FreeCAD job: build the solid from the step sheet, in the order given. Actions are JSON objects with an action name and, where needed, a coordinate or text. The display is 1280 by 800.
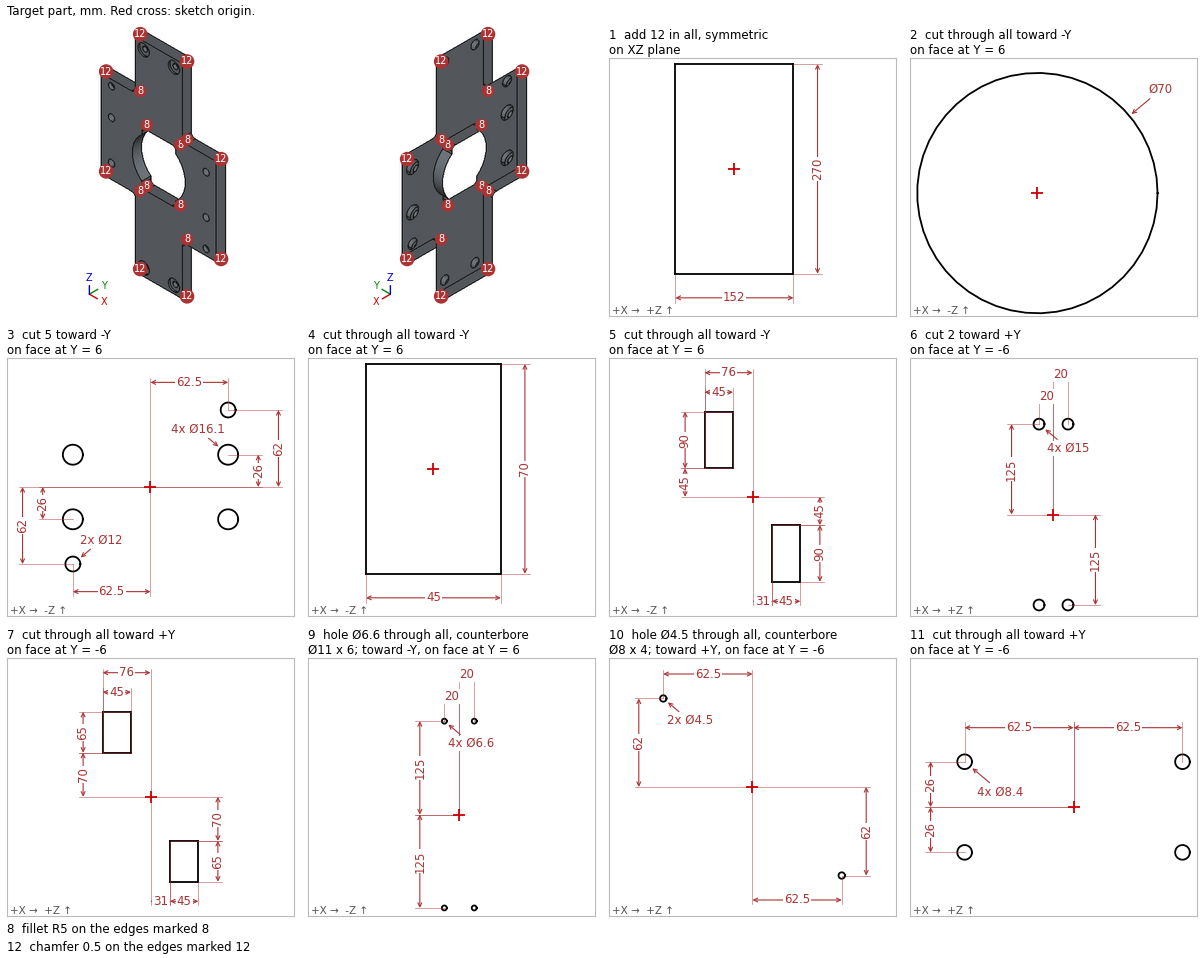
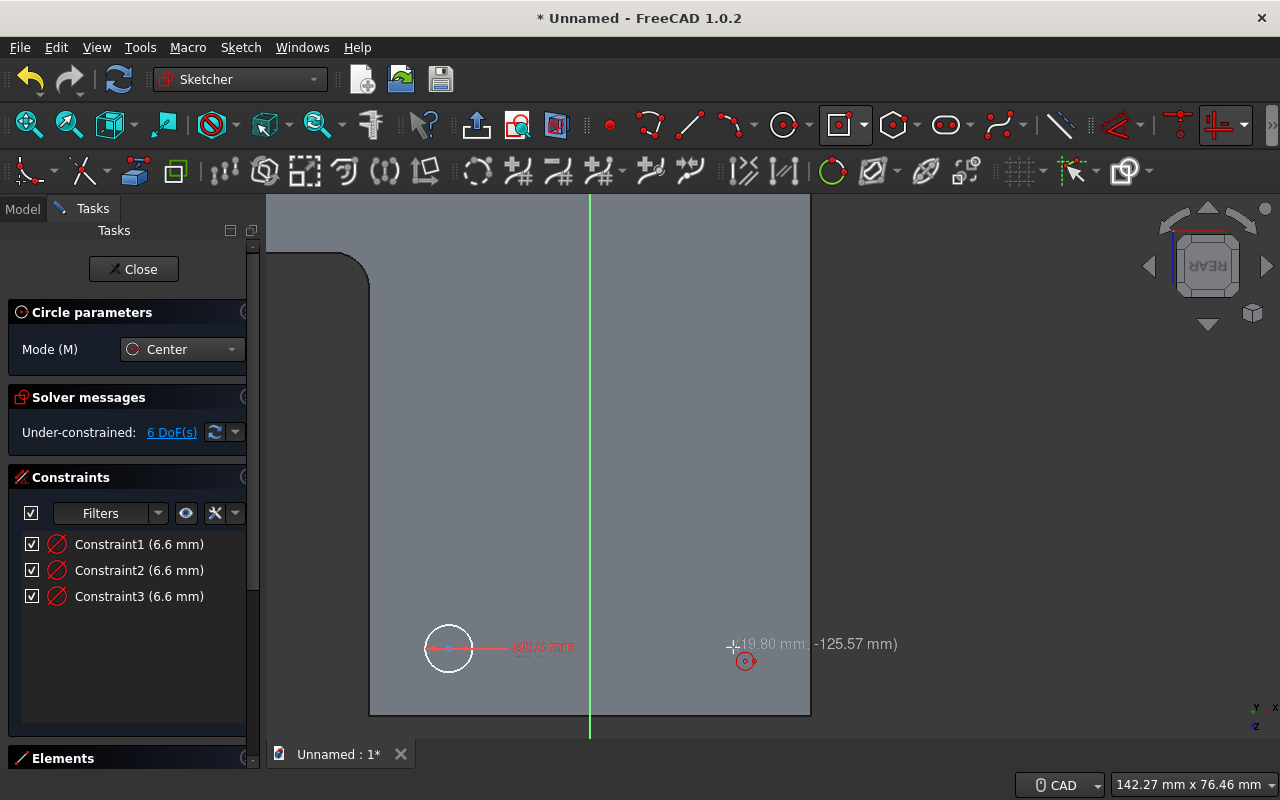
{"action": "scroll", "coordinate": [733, 647], "scroll_direction": "down", "scroll_amount": 8}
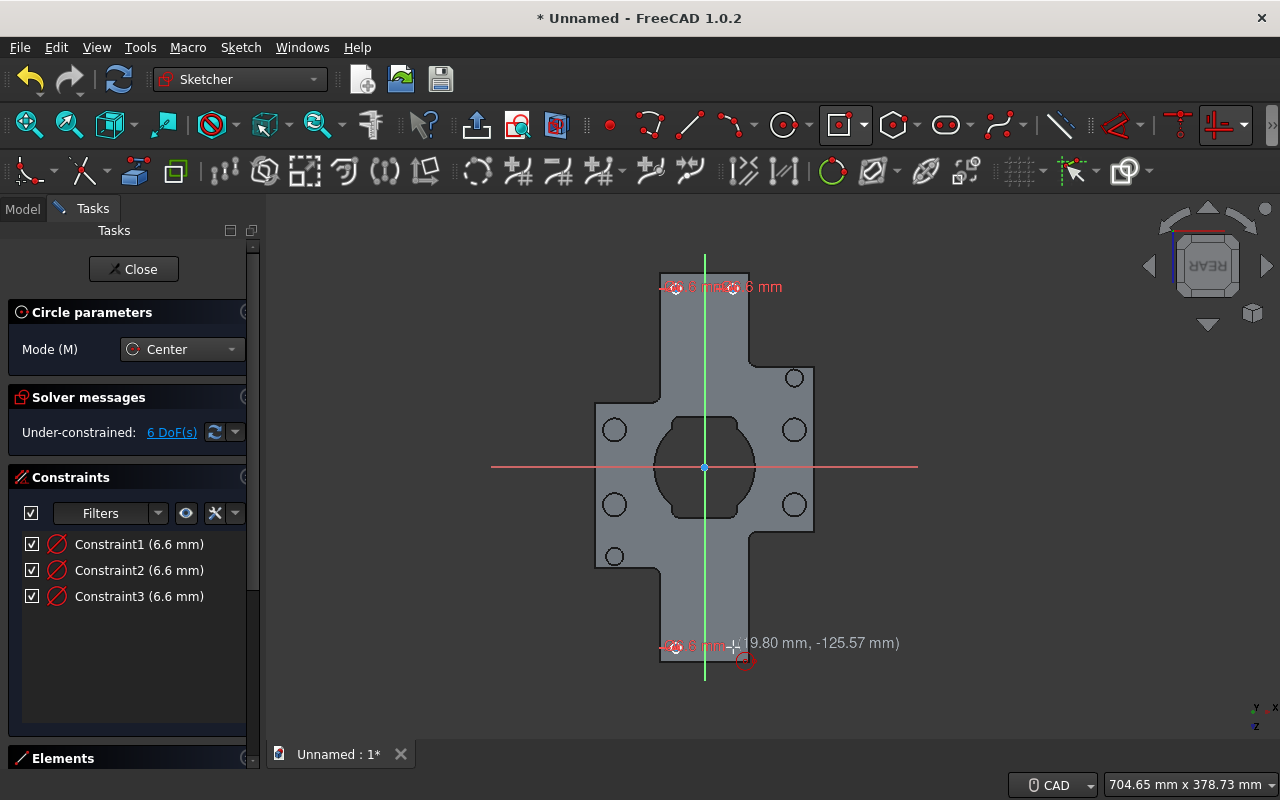
{"action": "left_click", "coordinate": [733, 647]}
{"action": "mouse_move", "coordinate": [737, 644]}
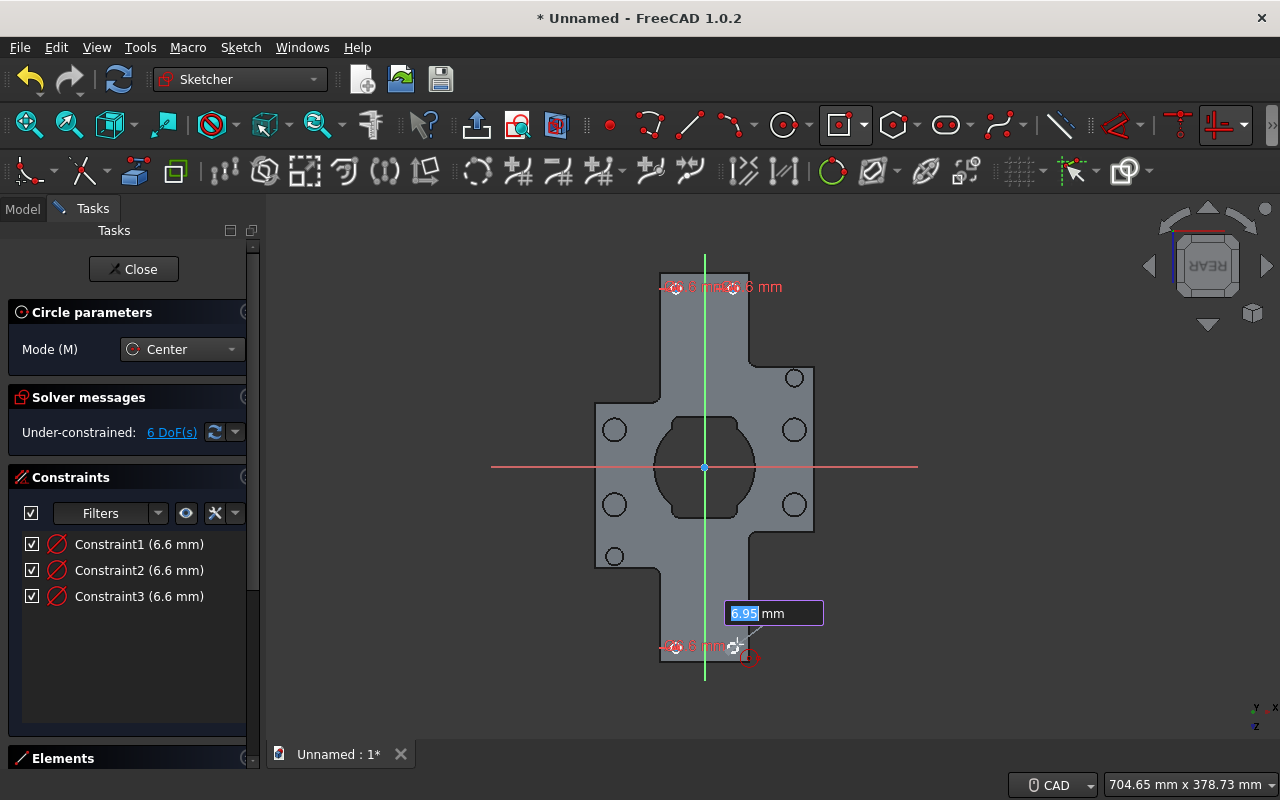
{"action": "type", "text": "6.6"}
{"action": "key", "text": "Return"}
{"action": "key", "text": "Escape"}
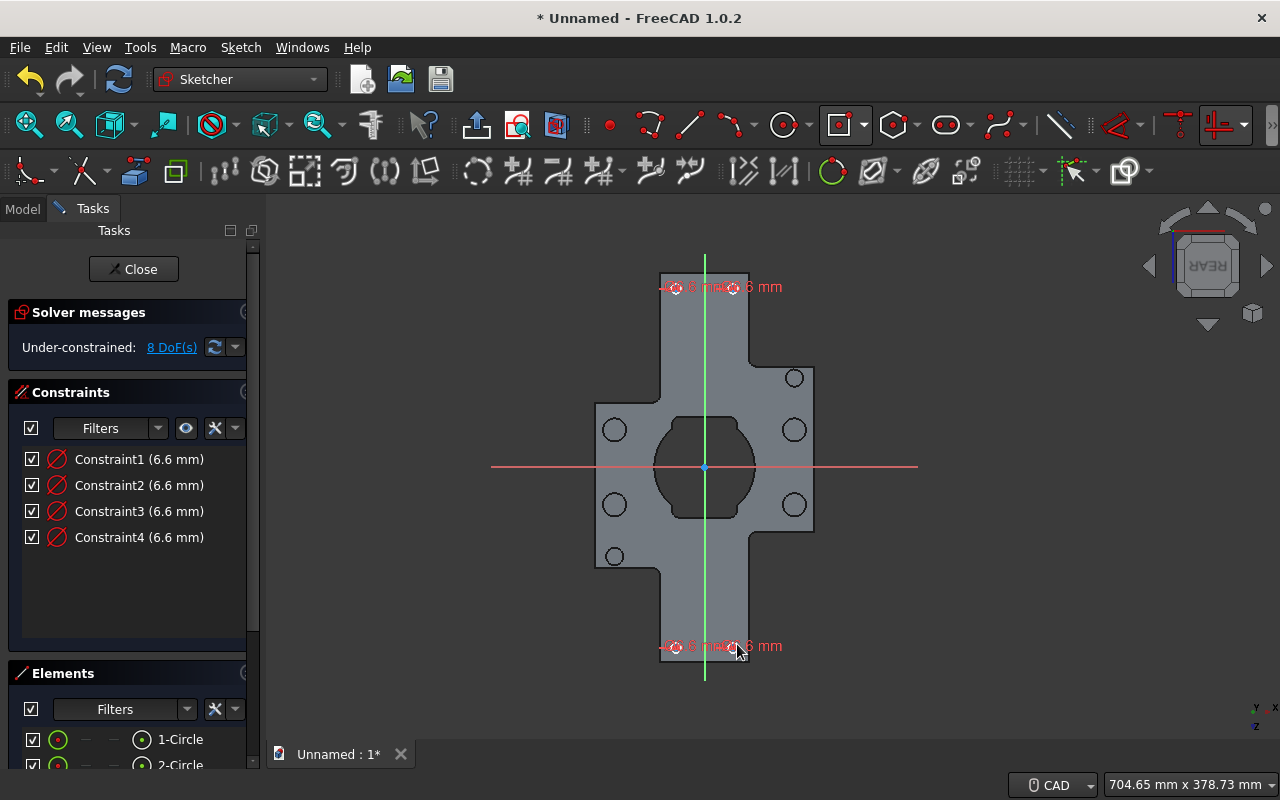
{"action": "left_click", "coordinate": [676, 289]}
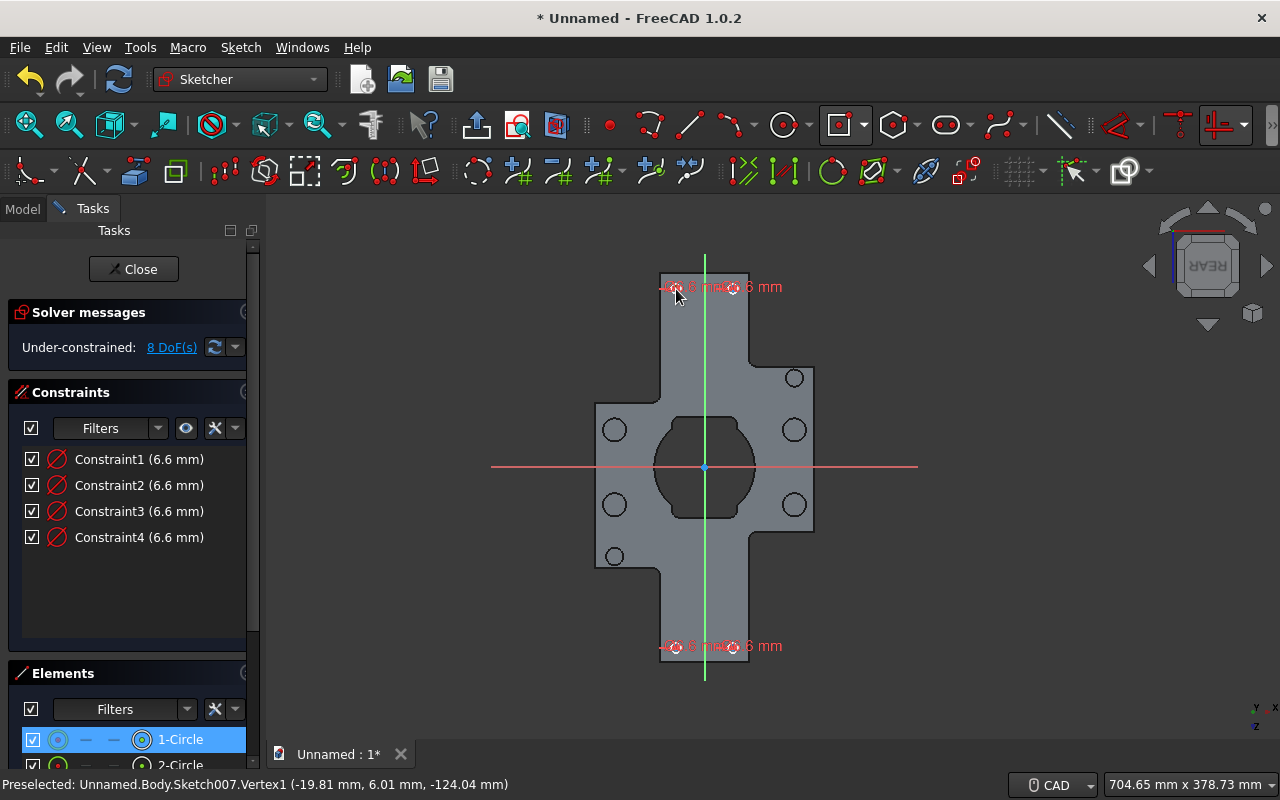
{"action": "left_click", "coordinate": [733, 289]}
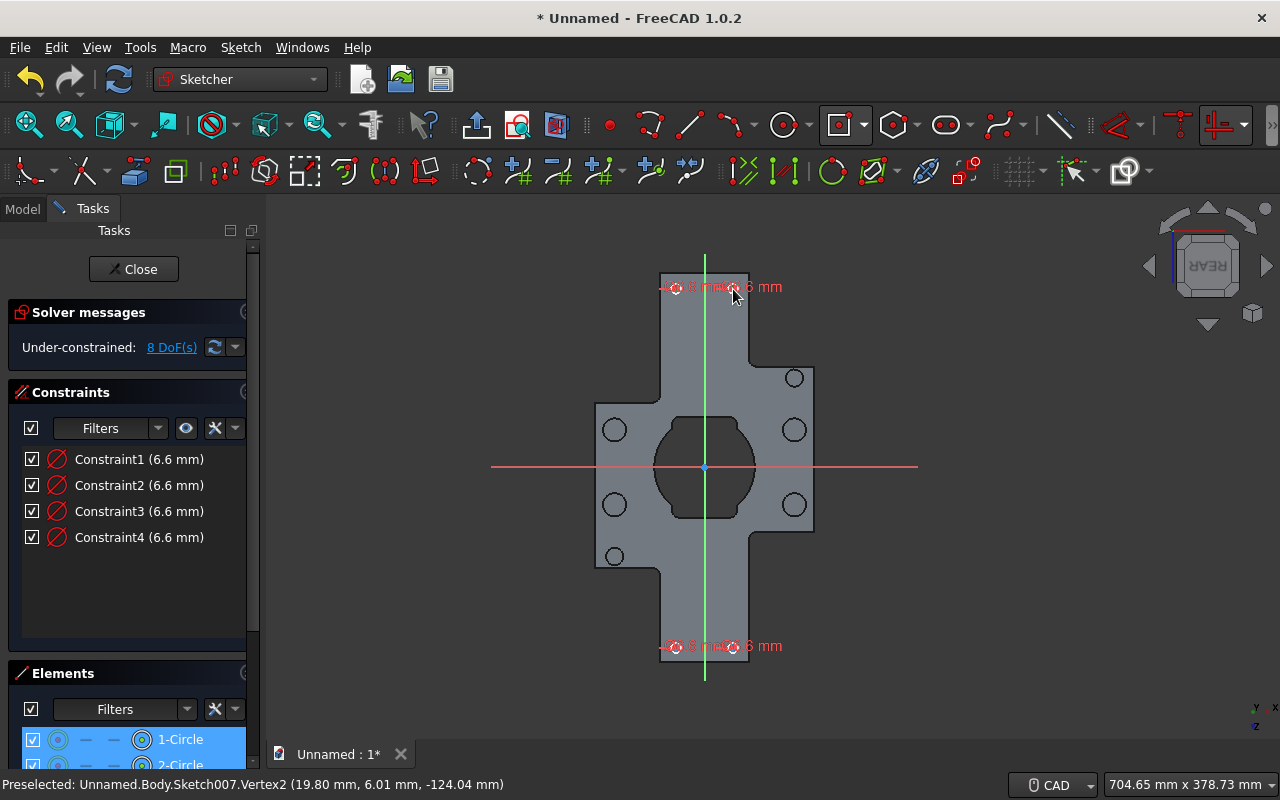
{"action": "key", "text": "h"}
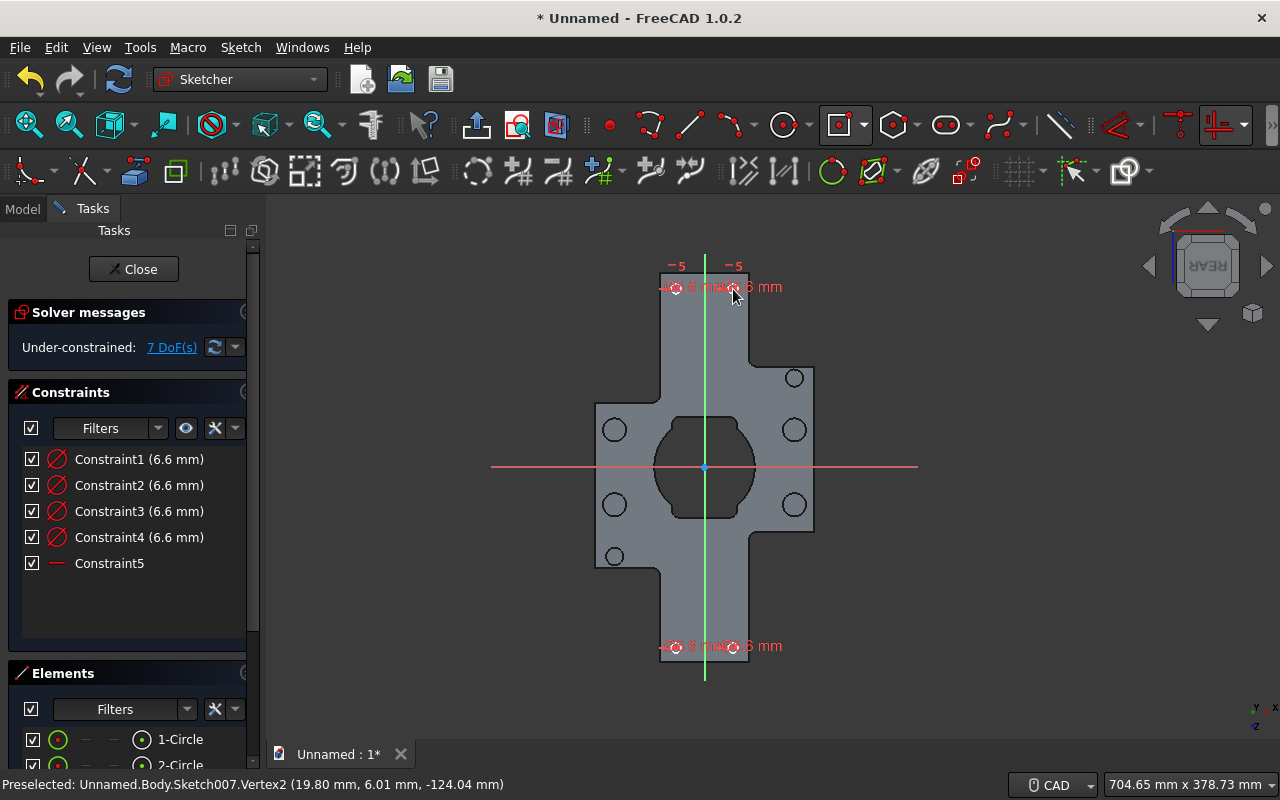
{"action": "left_click", "coordinate": [676, 289]}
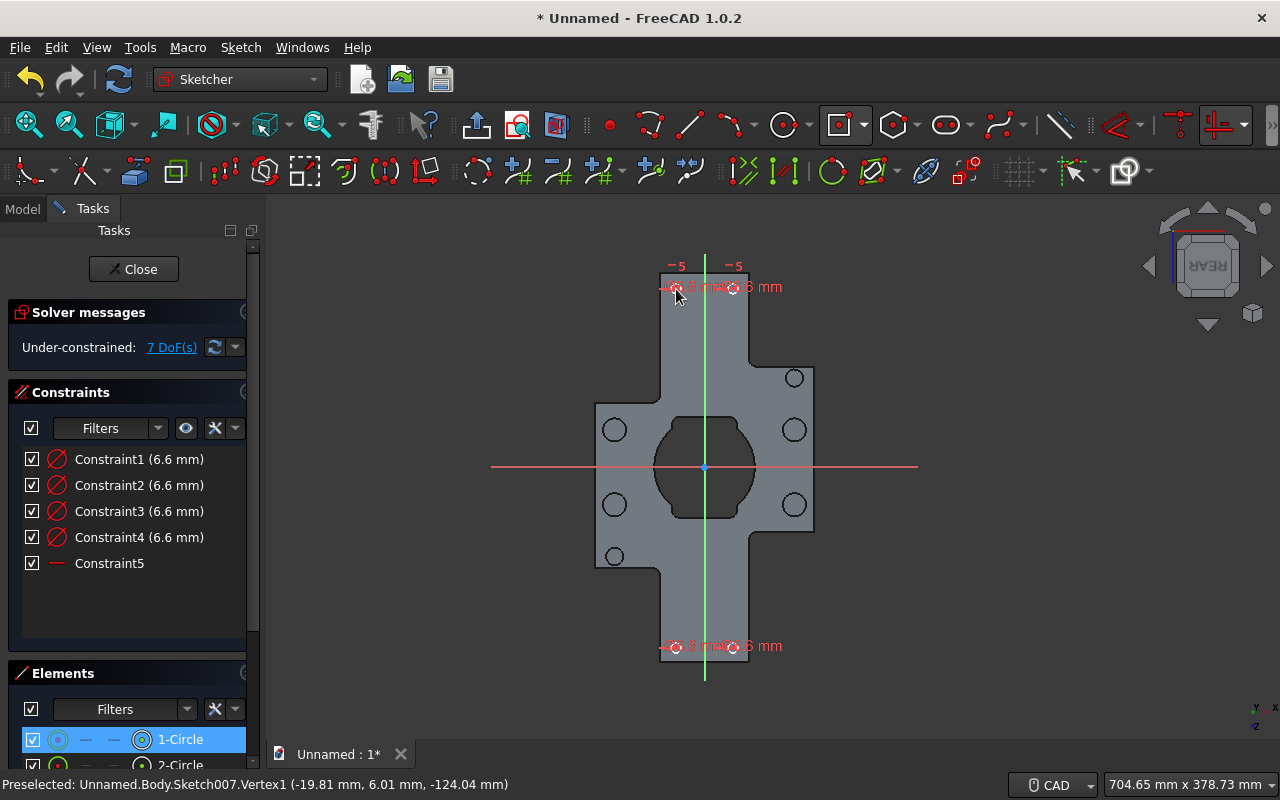
{"action": "left_click", "coordinate": [676, 648]}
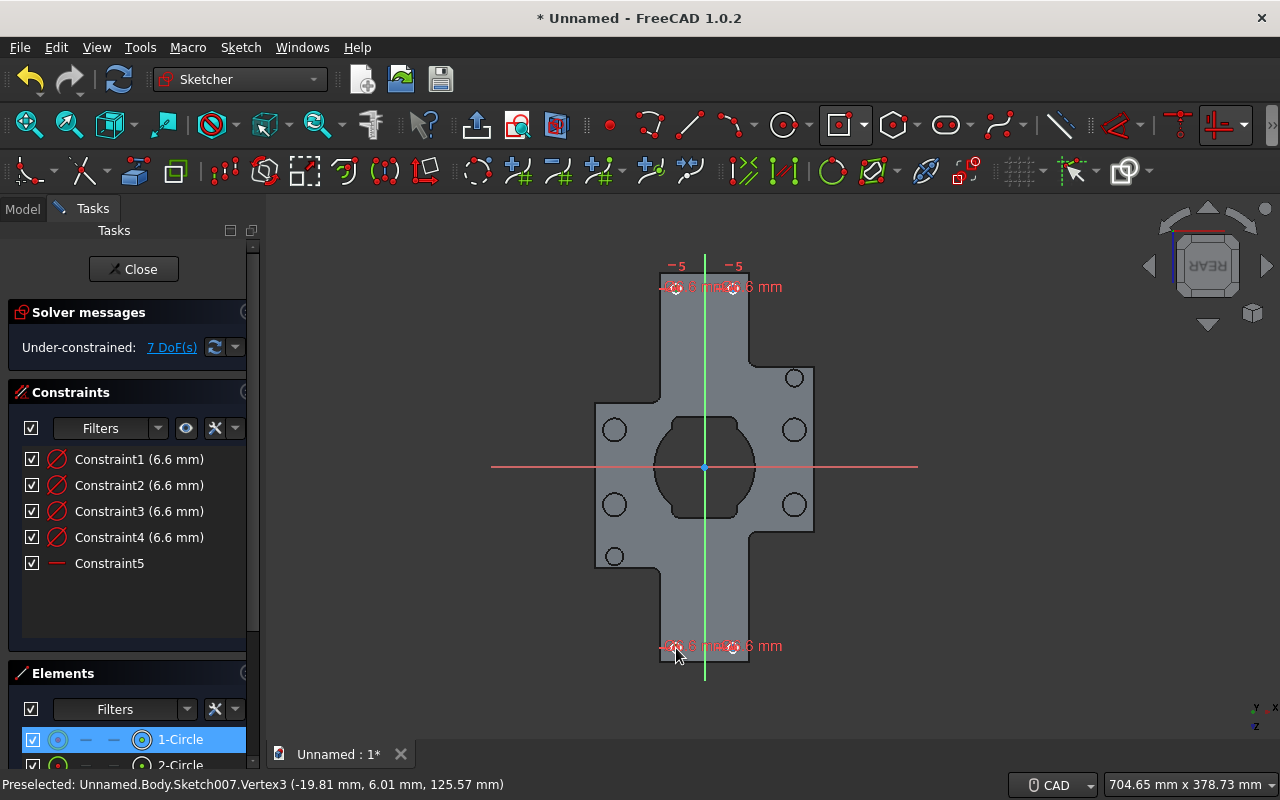
{"action": "key", "text": "v"}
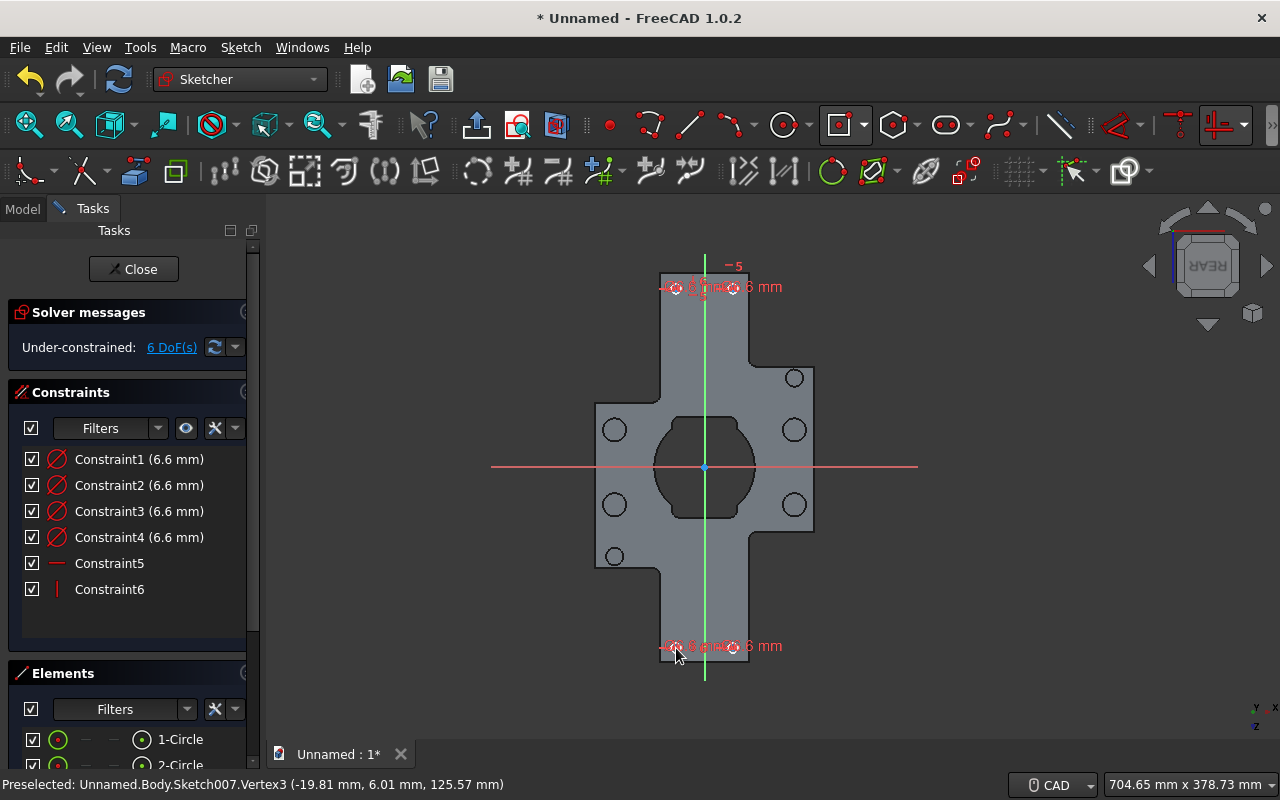
{"action": "left_click", "coordinate": [733, 289]}